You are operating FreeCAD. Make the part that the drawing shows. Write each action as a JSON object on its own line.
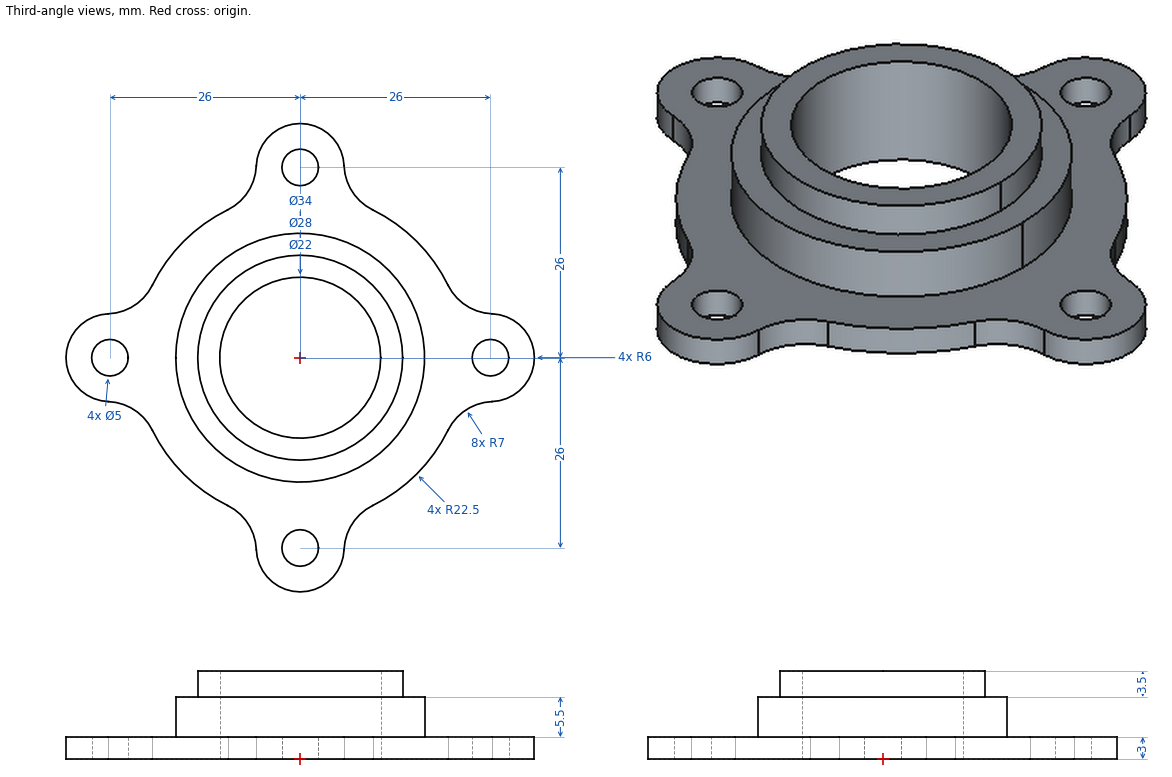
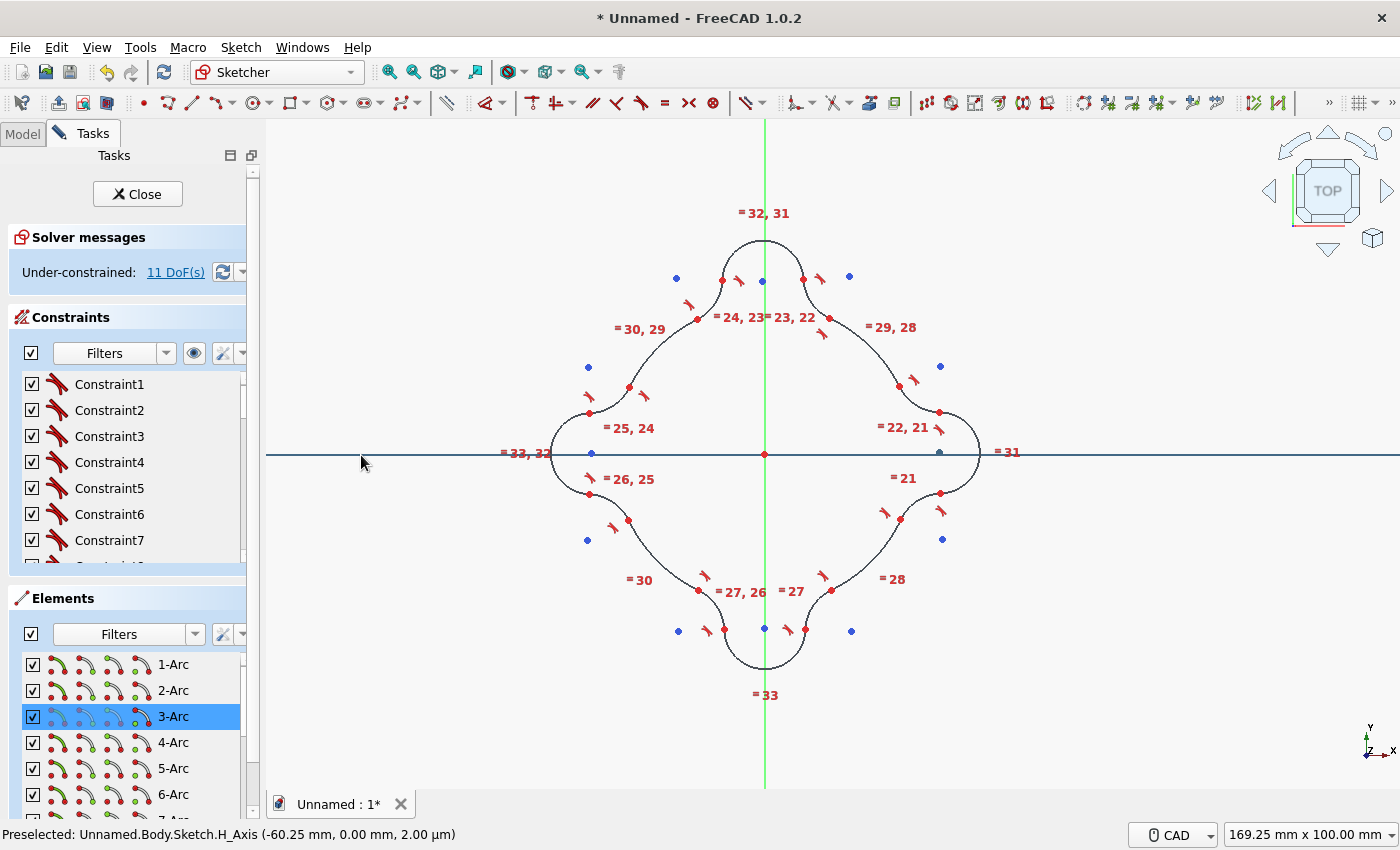
{"action": "left_click", "coordinate": [532, 104]}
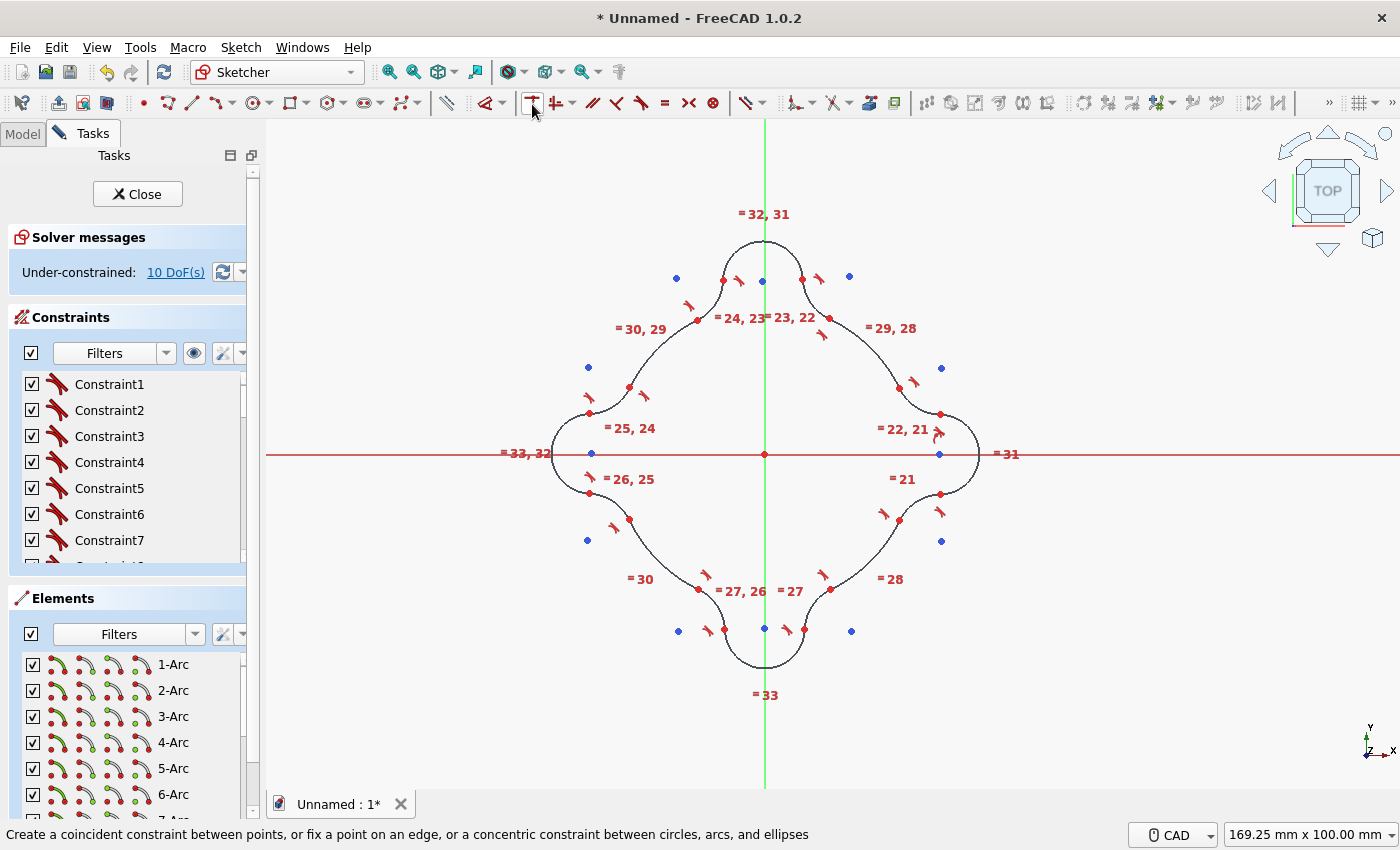
{"action": "left_click", "coordinate": [763, 281]}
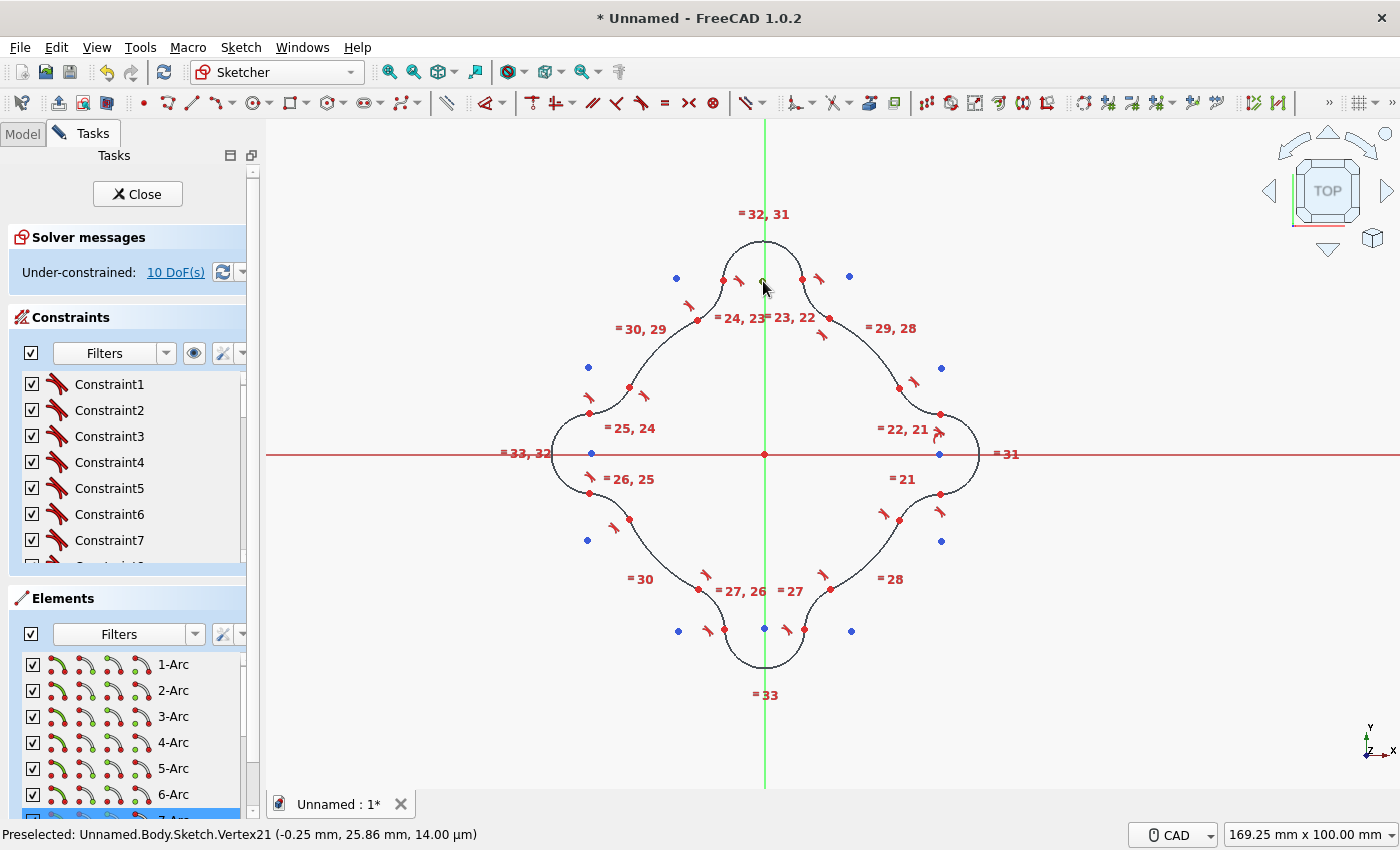
{"action": "left_click", "coordinate": [765, 717]}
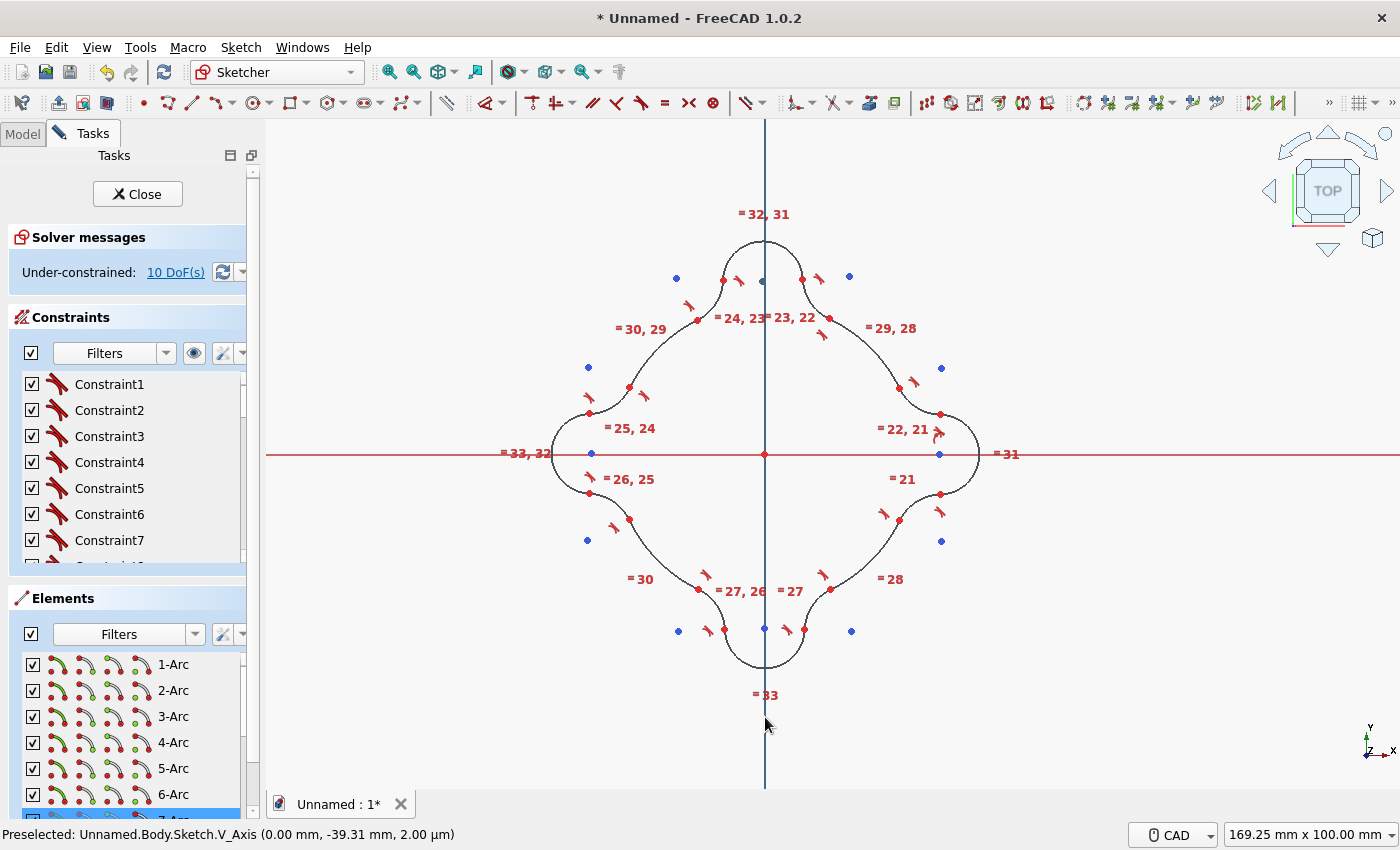
{"action": "left_click", "coordinate": [532, 104]}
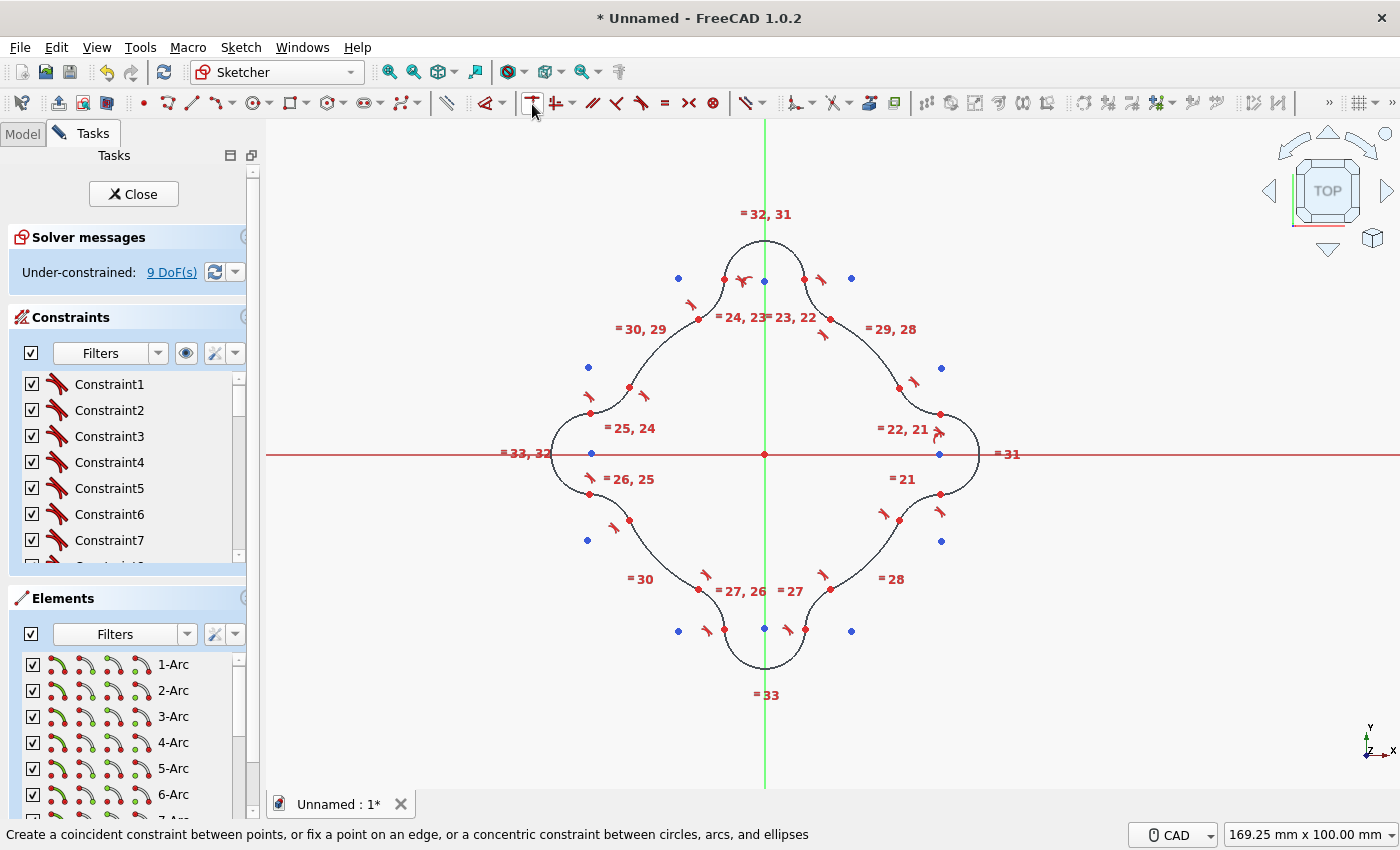
{"action": "left_click", "coordinate": [591, 454]}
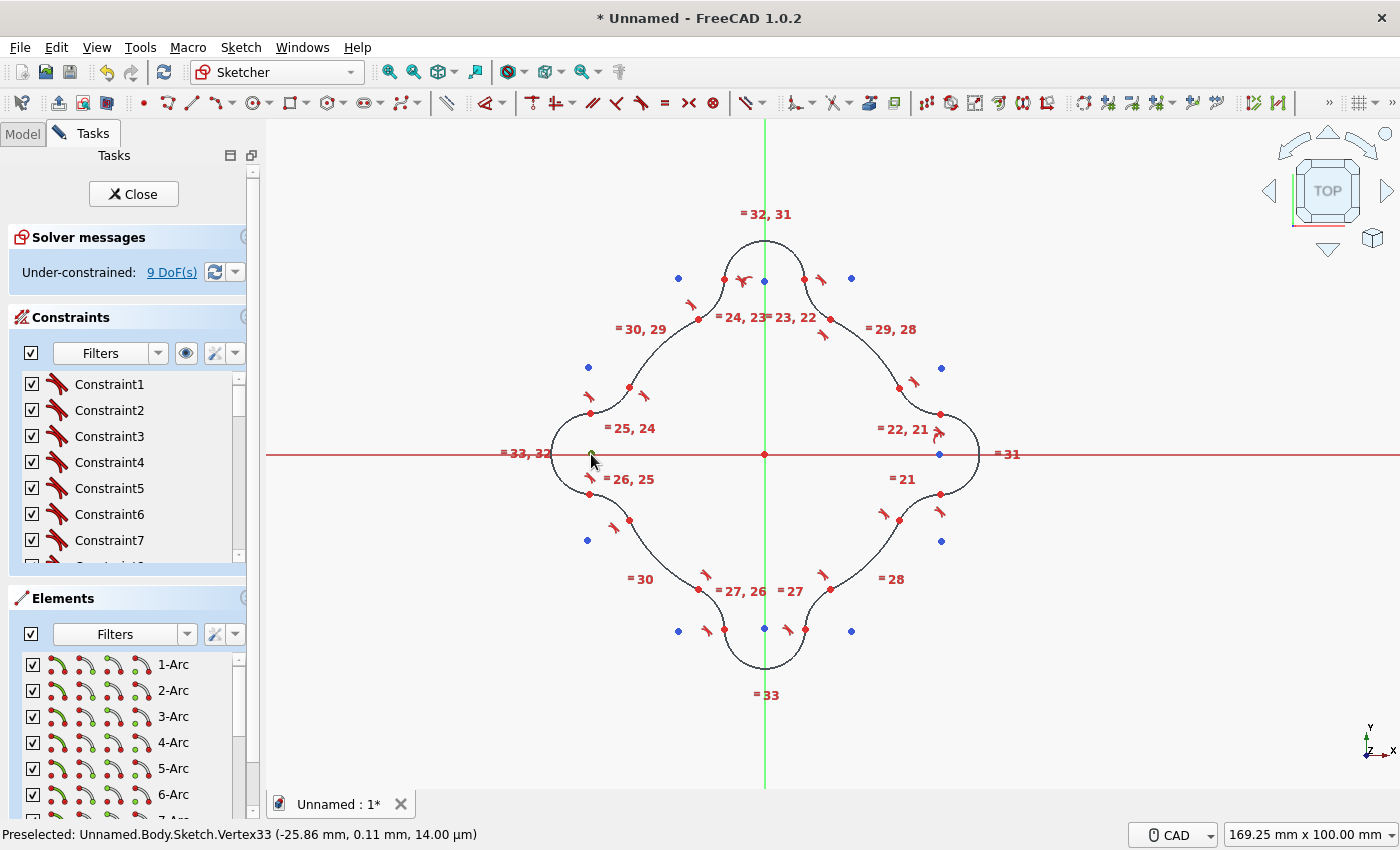
{"action": "left_click", "coordinate": [361, 455]}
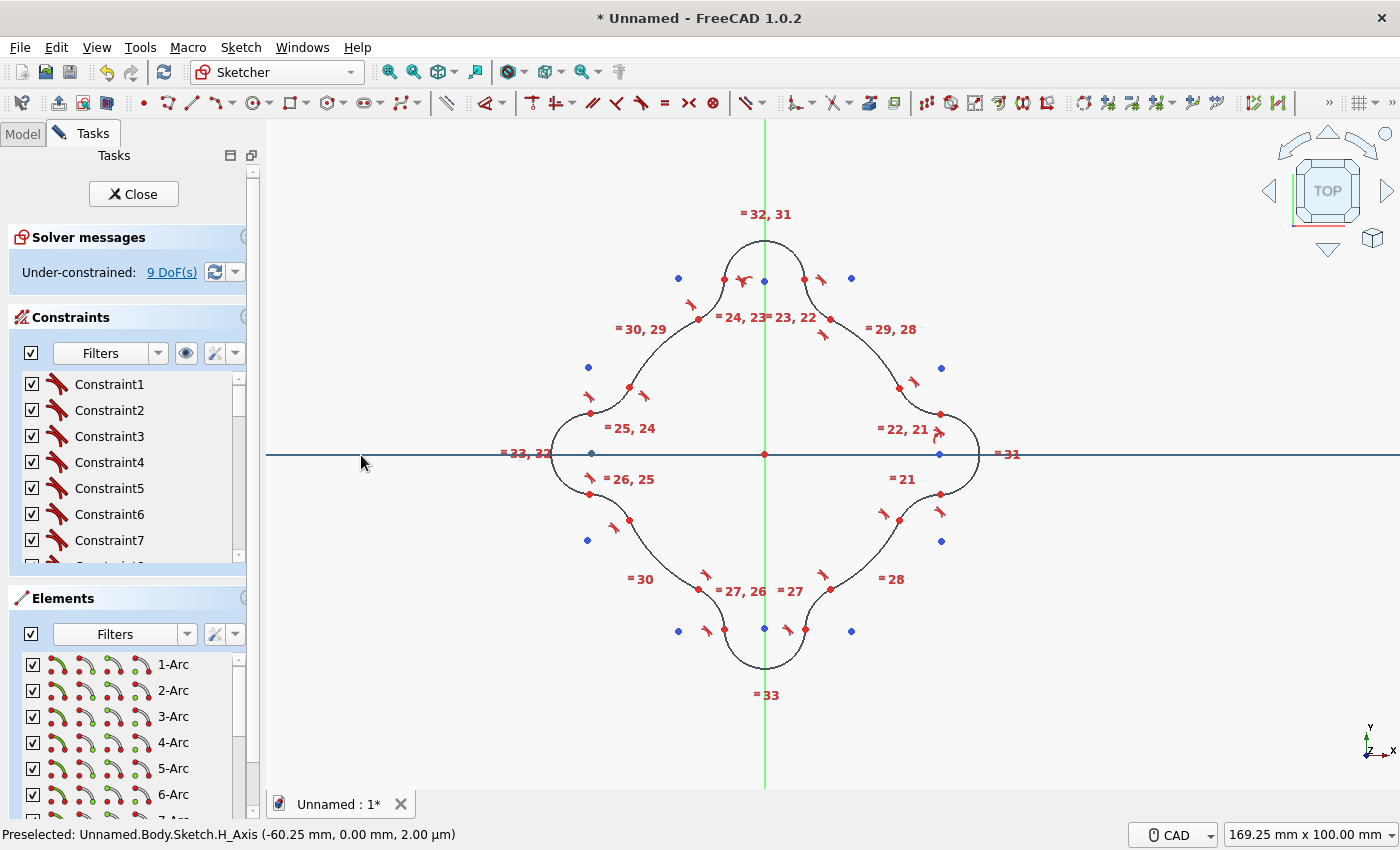
{"action": "left_click", "coordinate": [532, 104]}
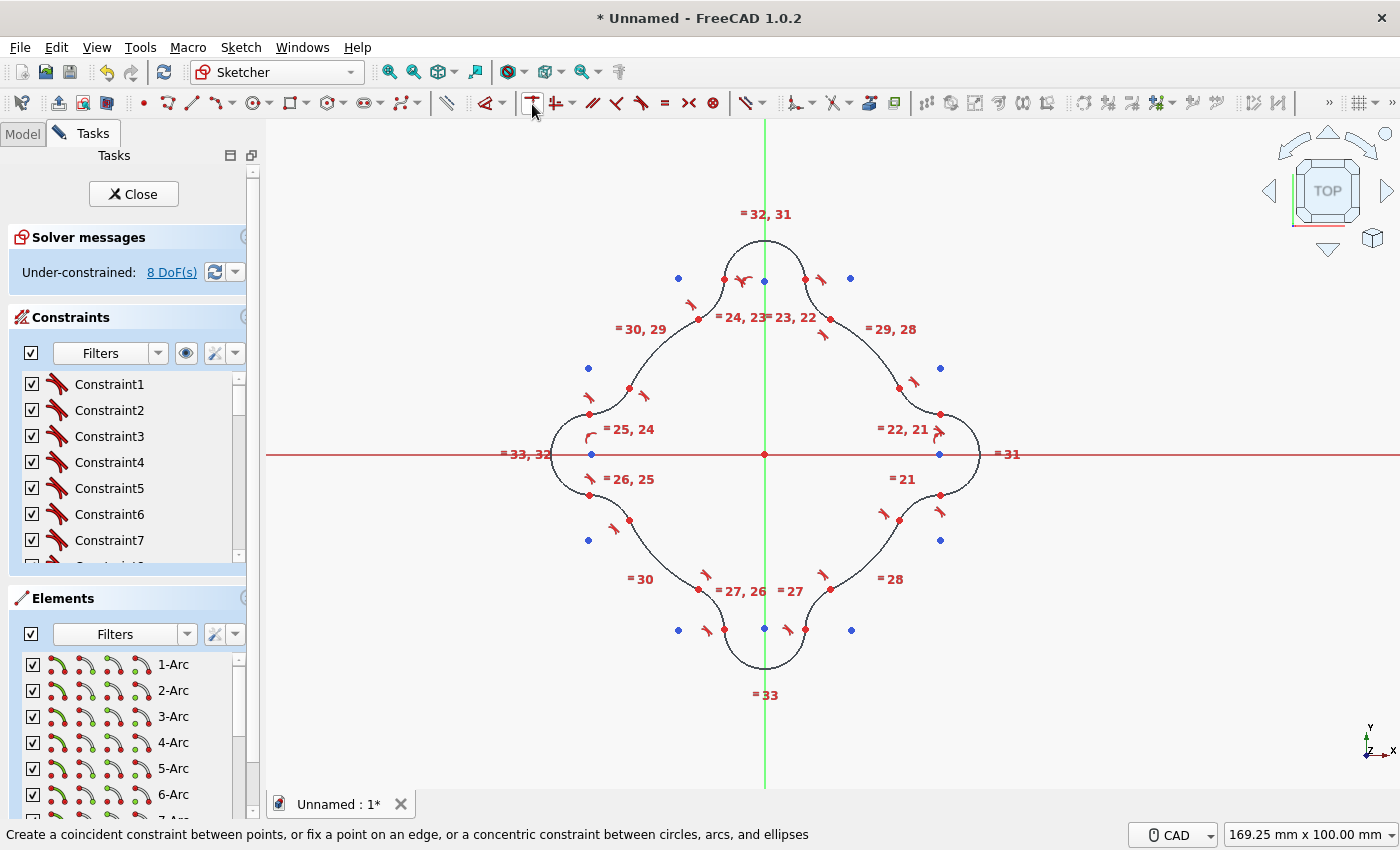
{"action": "left_click", "coordinate": [765, 629]}